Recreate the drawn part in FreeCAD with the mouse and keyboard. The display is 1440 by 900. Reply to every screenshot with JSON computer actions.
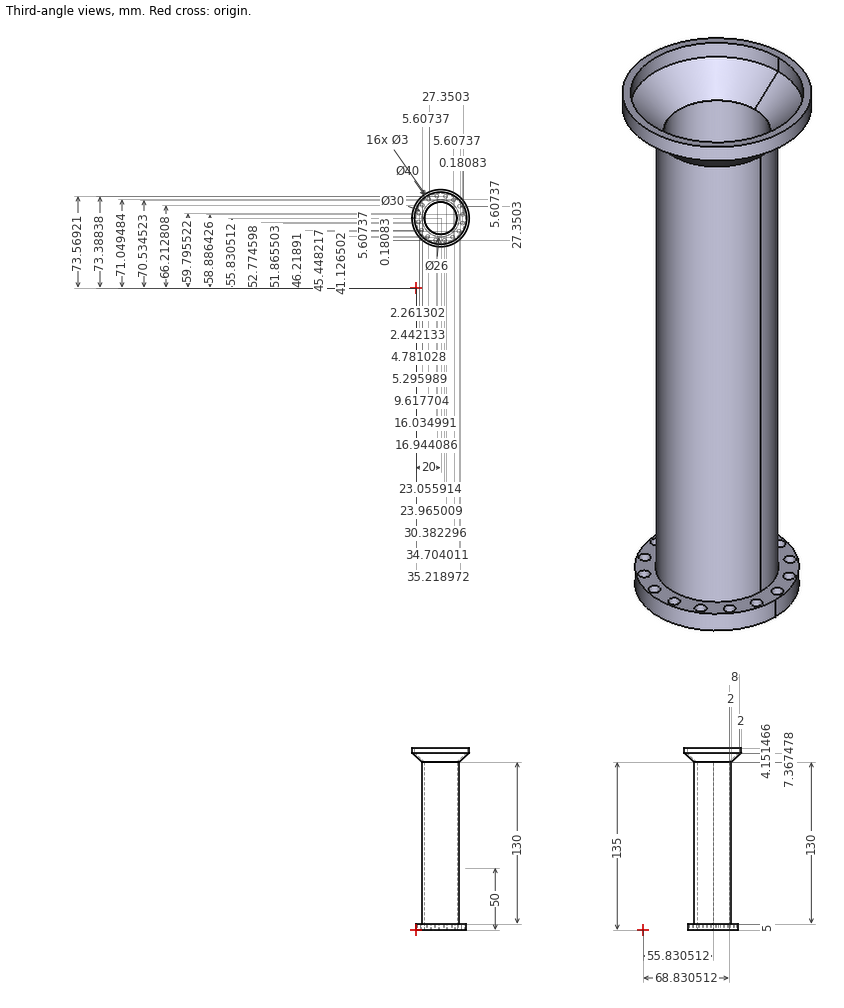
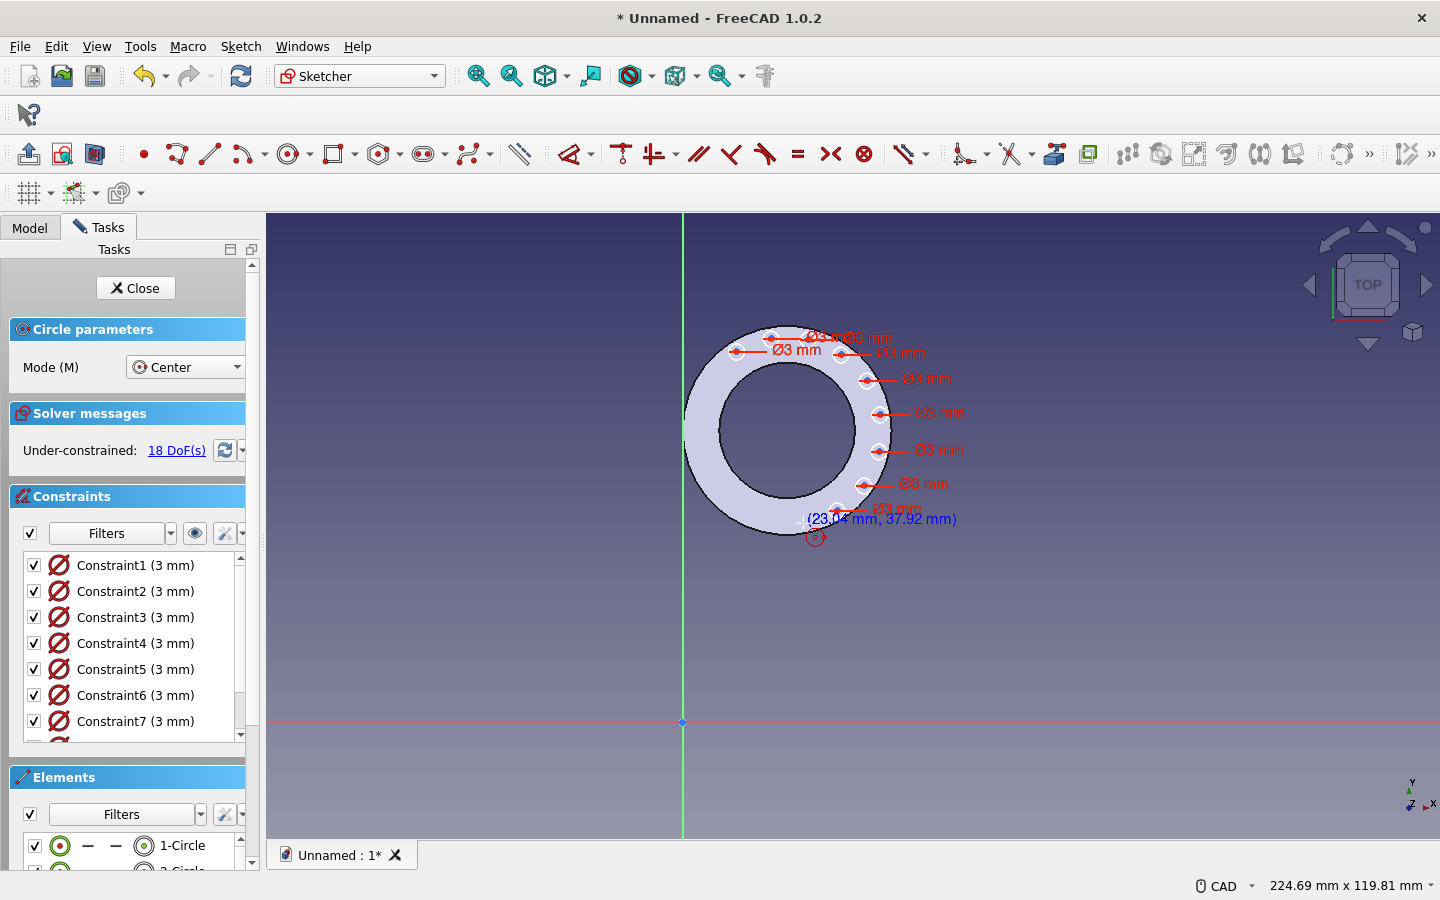
{"action": "left_click", "coordinate": [803, 523]}
{"action": "mouse_move", "coordinate": [809, 518]}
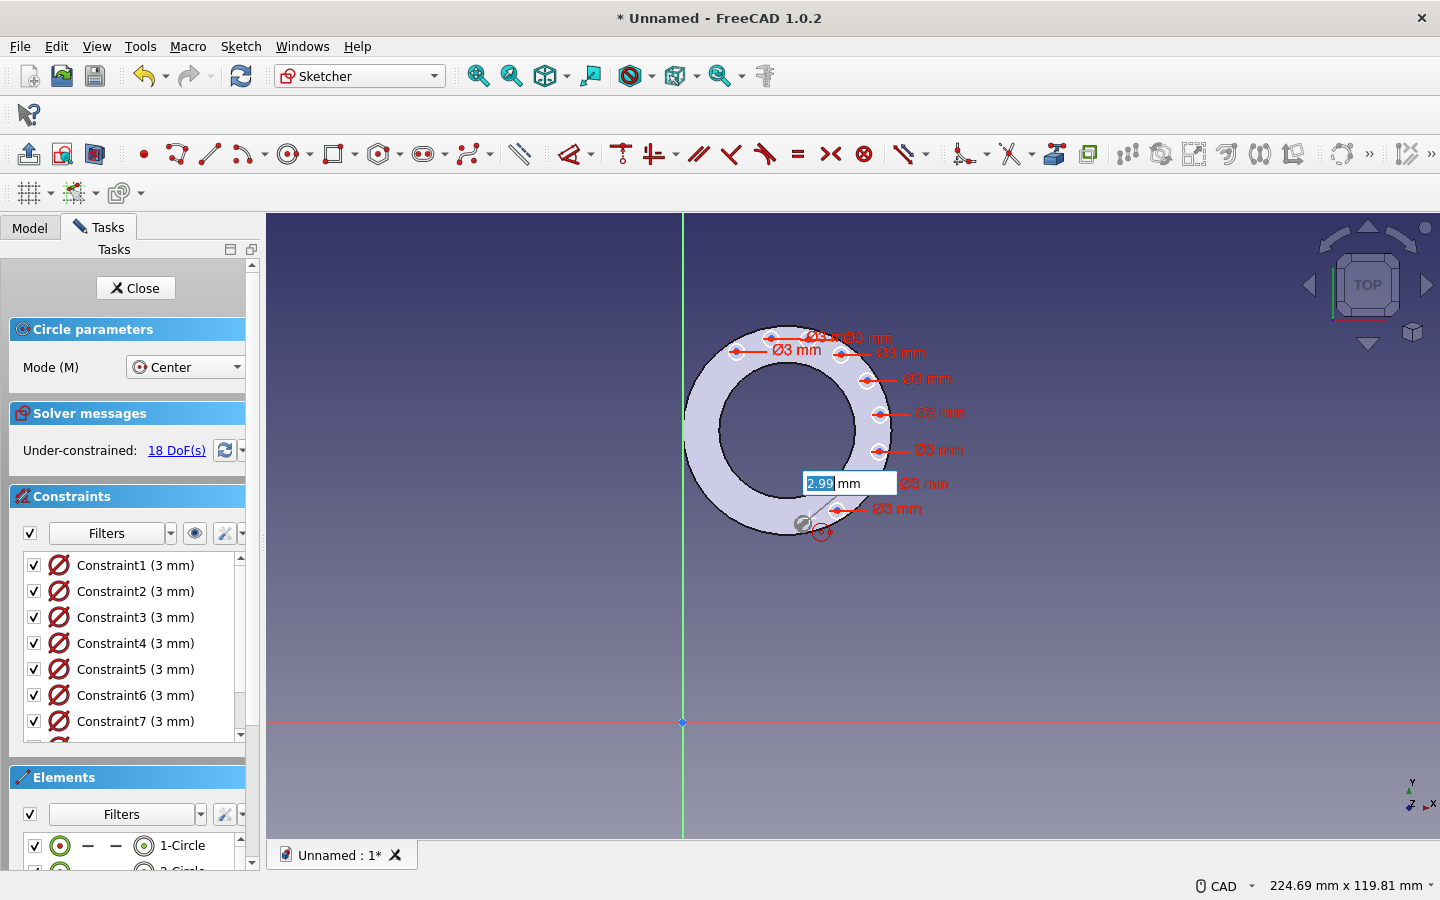
{"action": "type", "text": "3"}
{"action": "key", "text": "Return"}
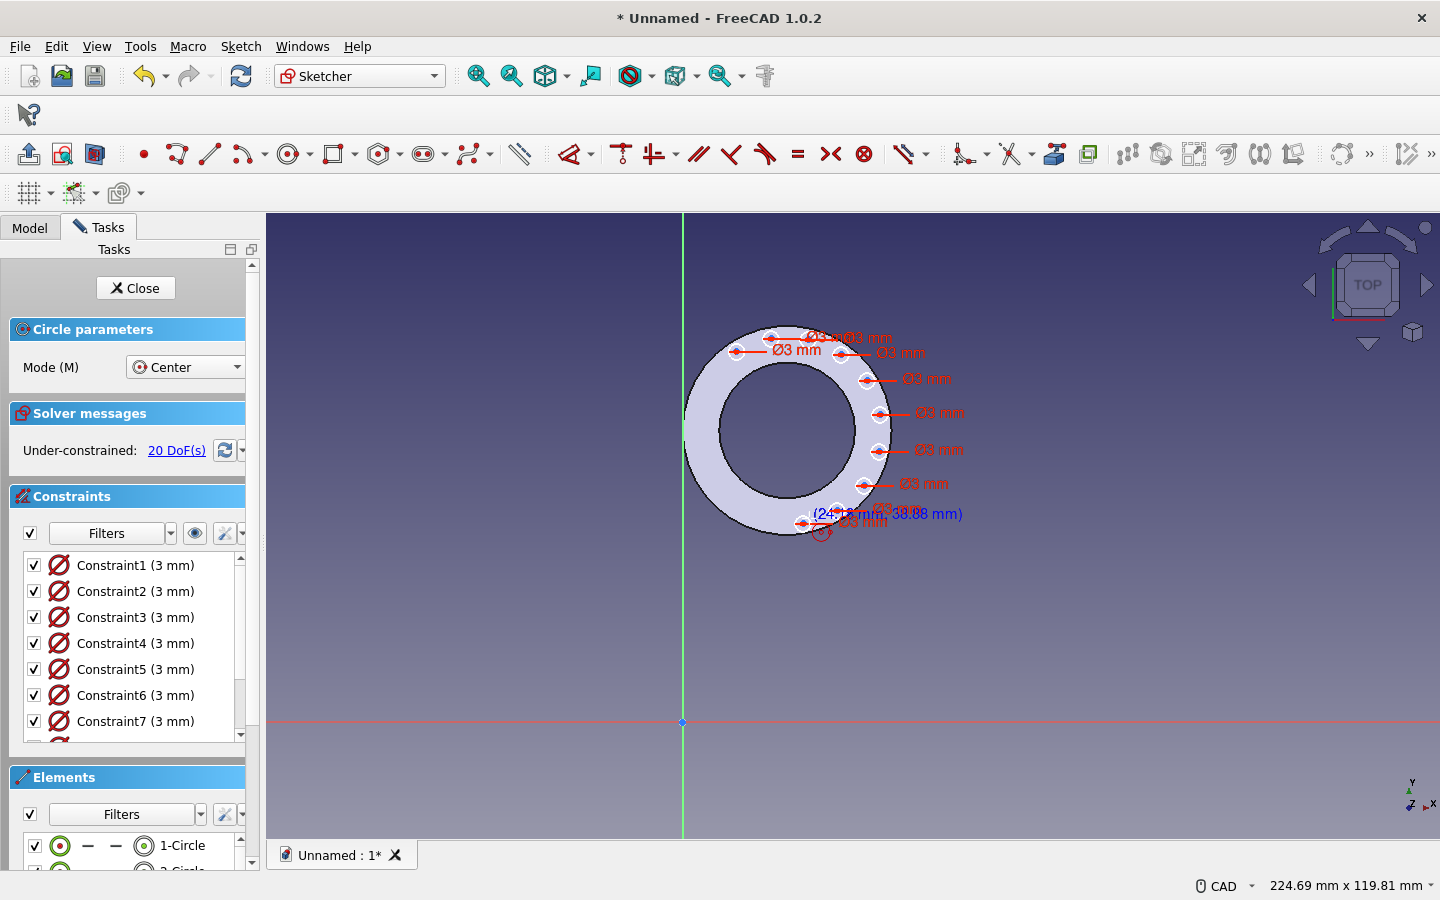
{"action": "scroll", "coordinate": [766, 522], "scroll_direction": "up", "scroll_amount": 6}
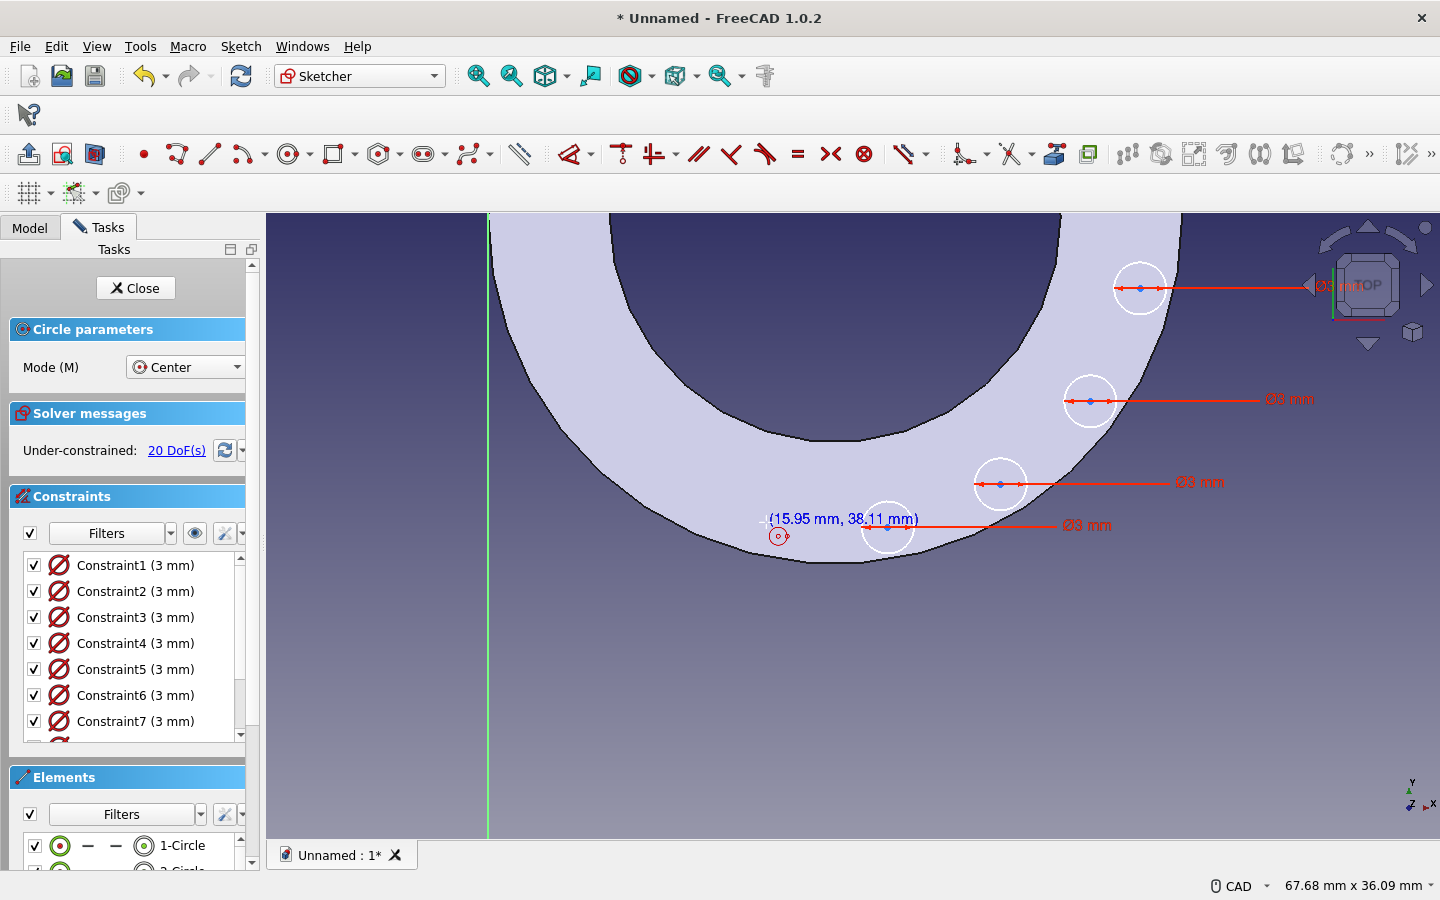
{"action": "scroll", "coordinate": [765, 522], "scroll_direction": "down", "scroll_amount": 6}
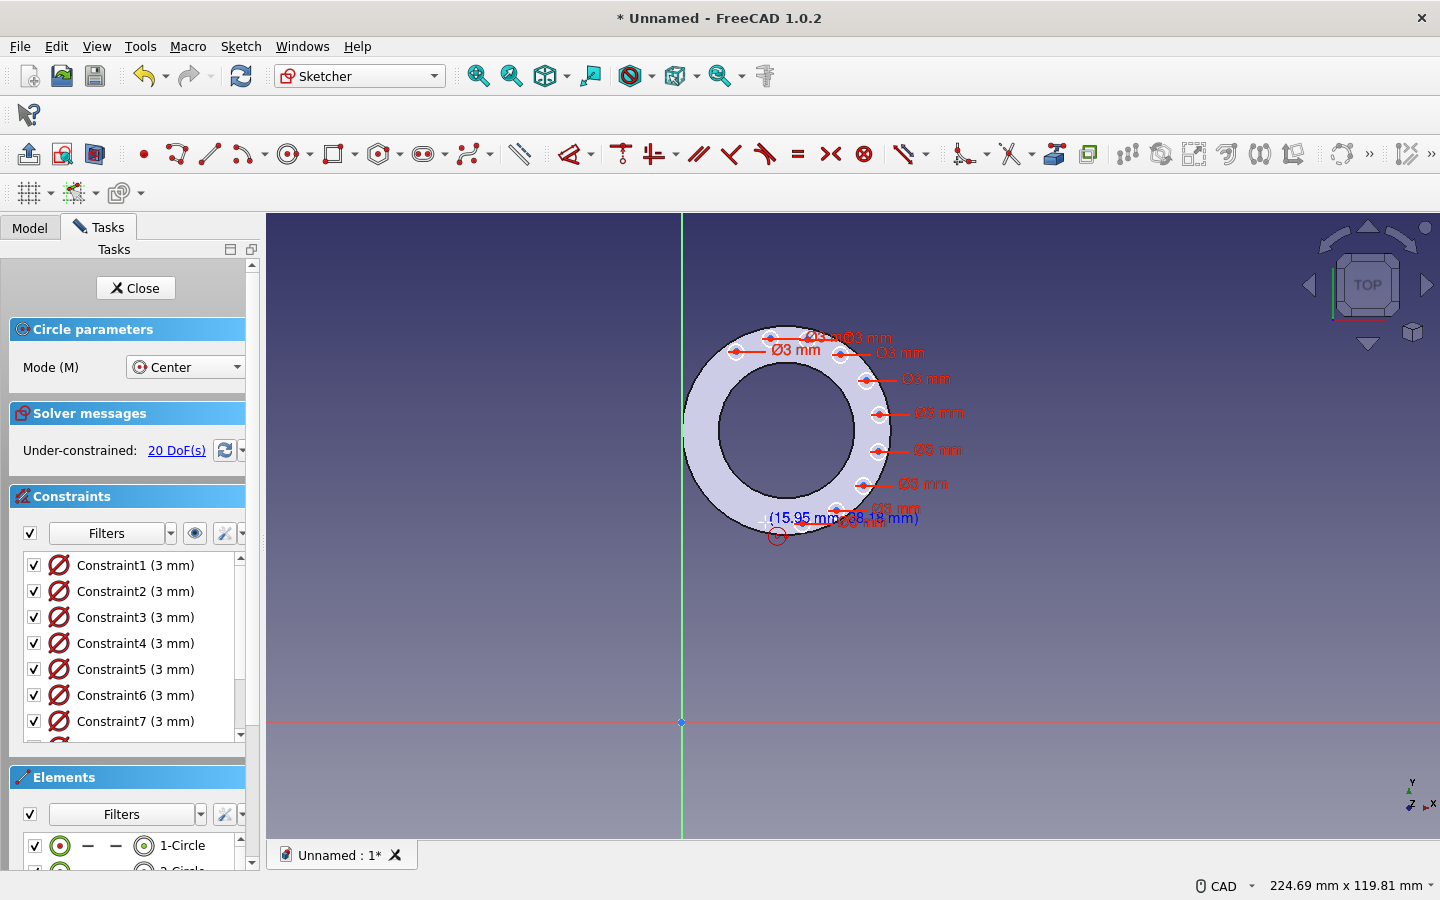
{"action": "left_click", "coordinate": [766, 522]}
{"action": "mouse_move", "coordinate": [771, 517]}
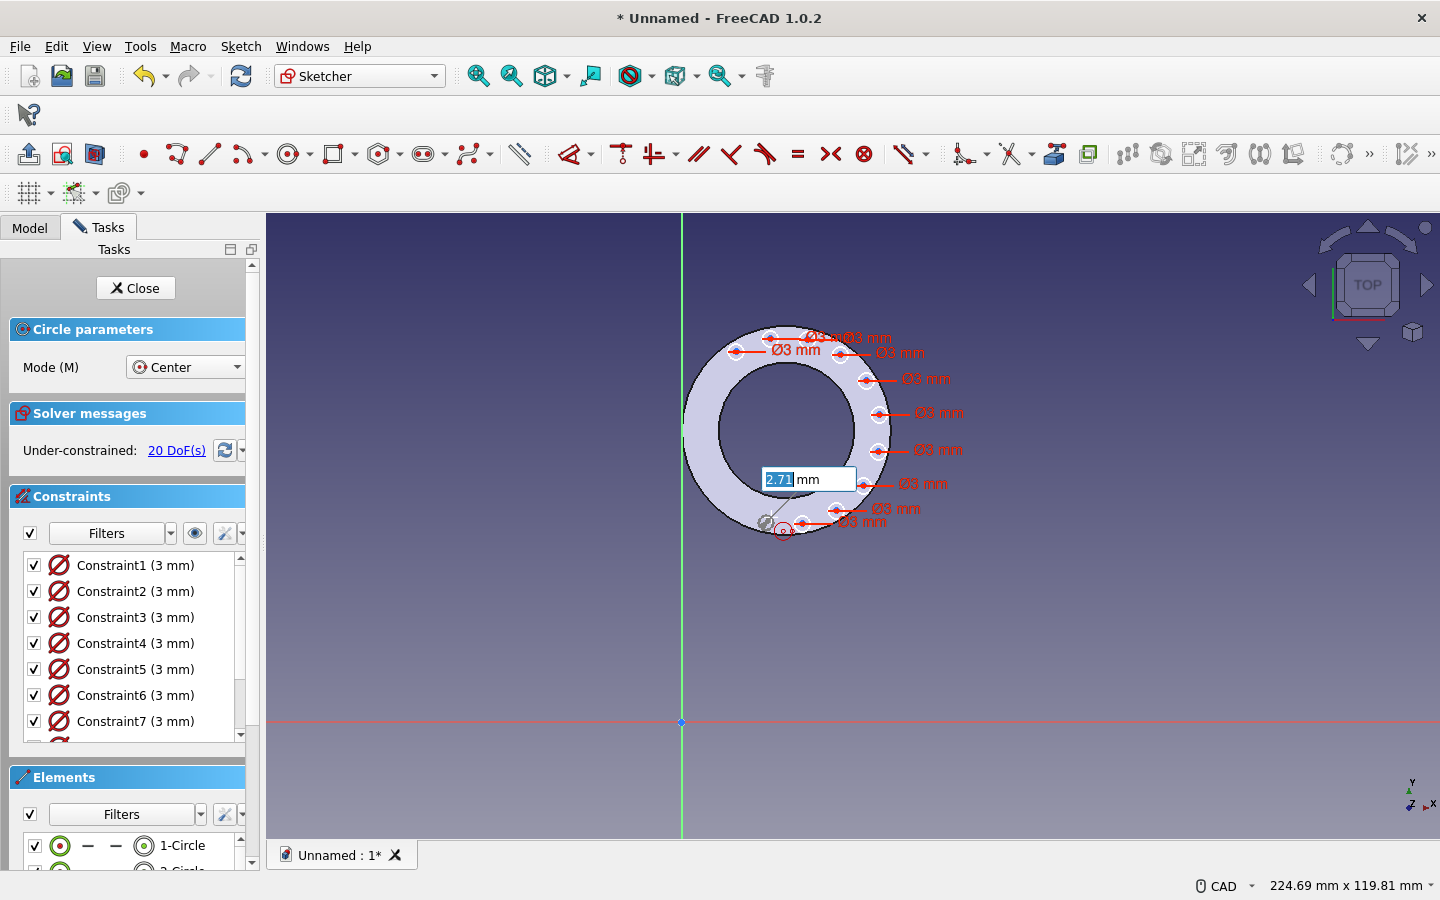
{"action": "type", "text": "3"}
{"action": "key", "text": "Return"}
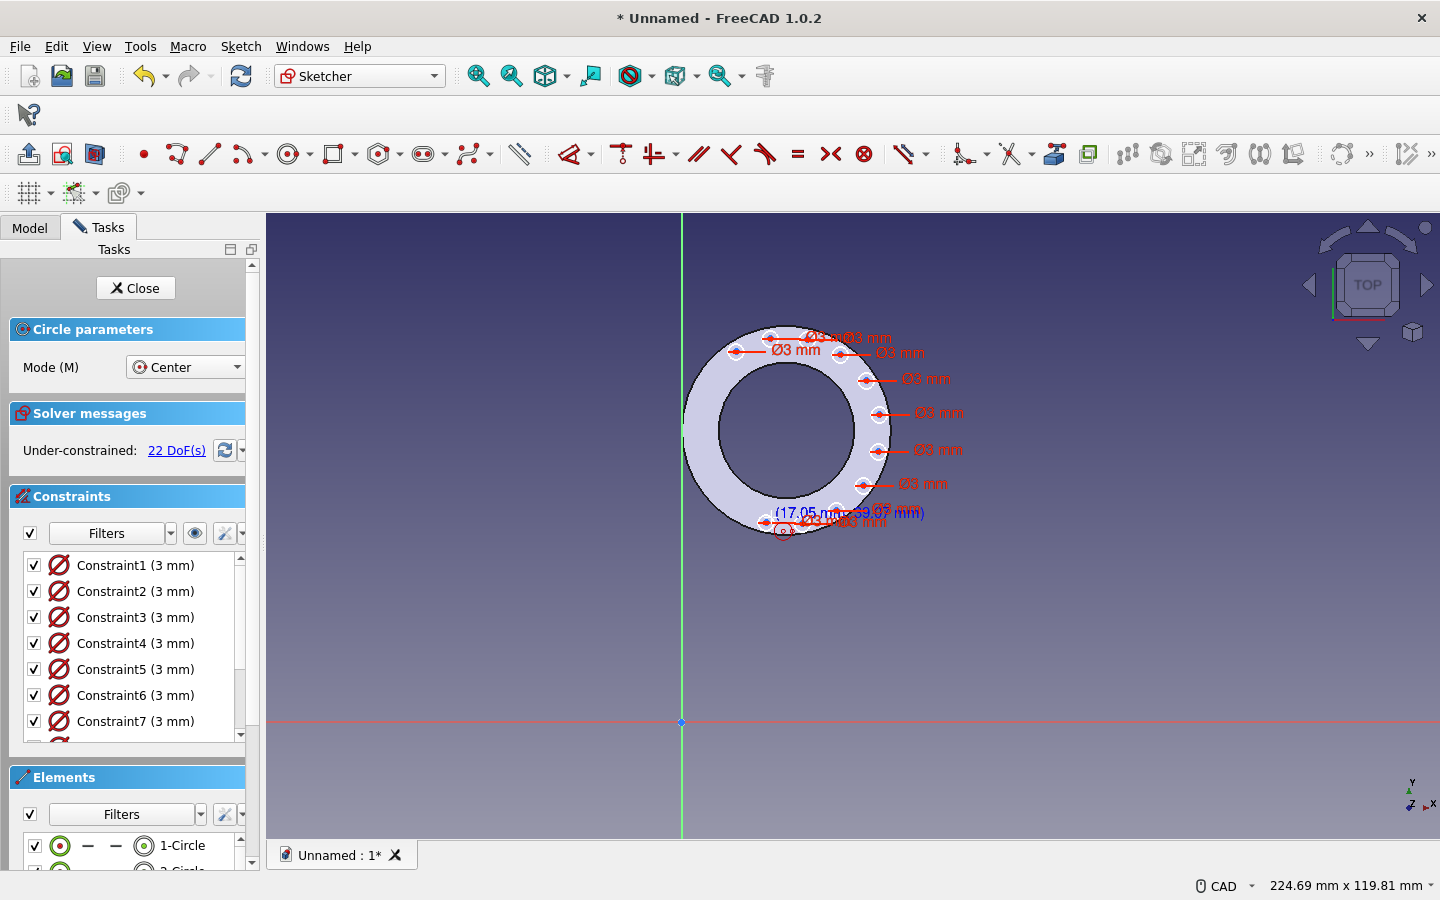
{"action": "scroll", "coordinate": [732, 507], "scroll_direction": "up", "scroll_amount": 6}